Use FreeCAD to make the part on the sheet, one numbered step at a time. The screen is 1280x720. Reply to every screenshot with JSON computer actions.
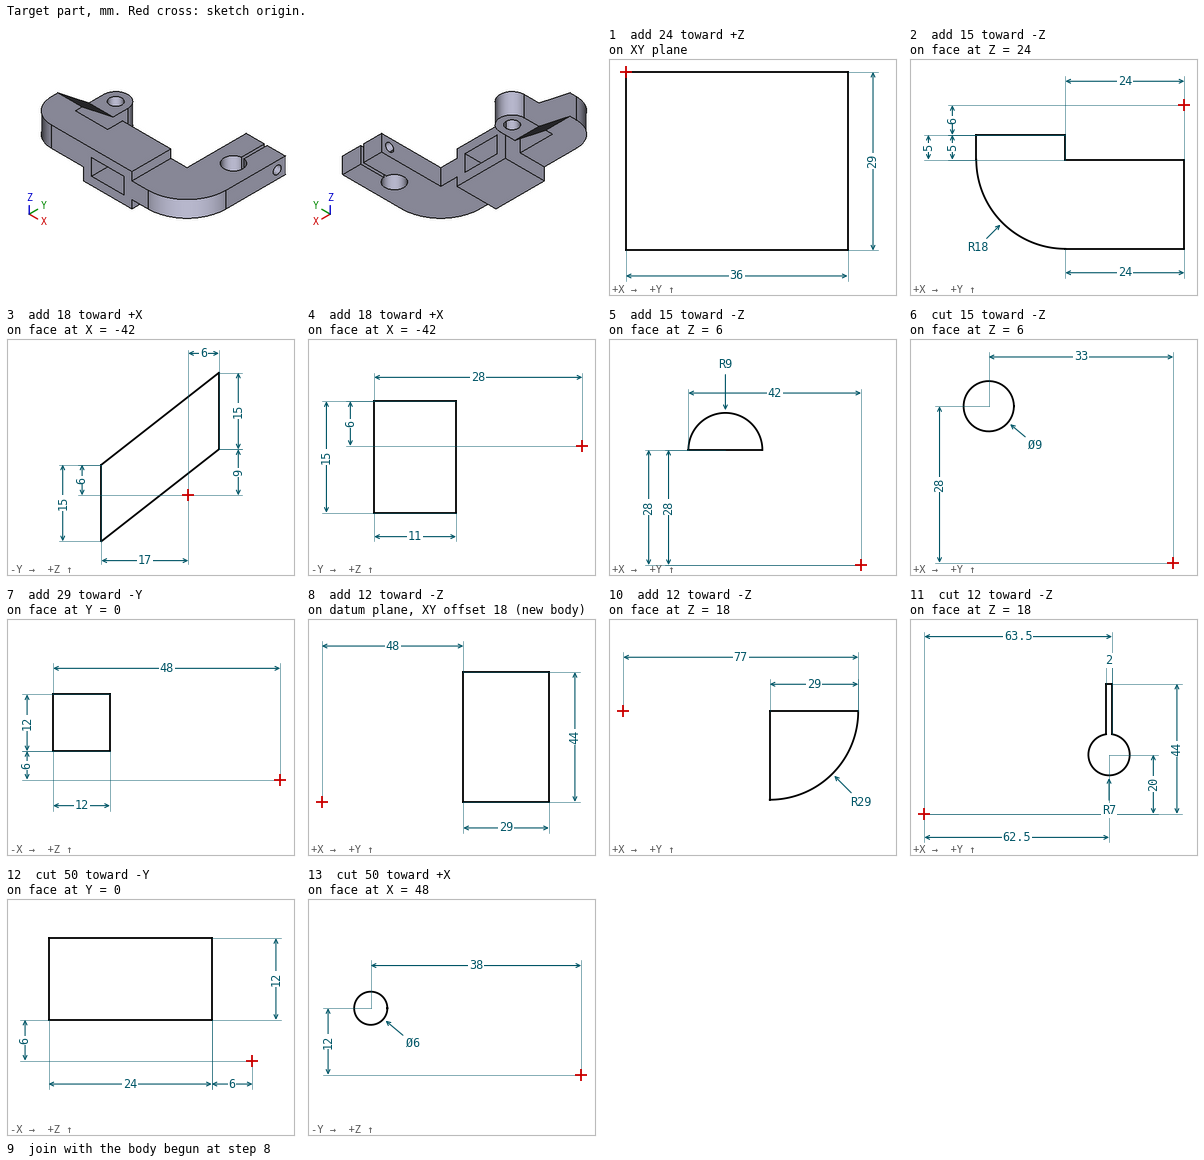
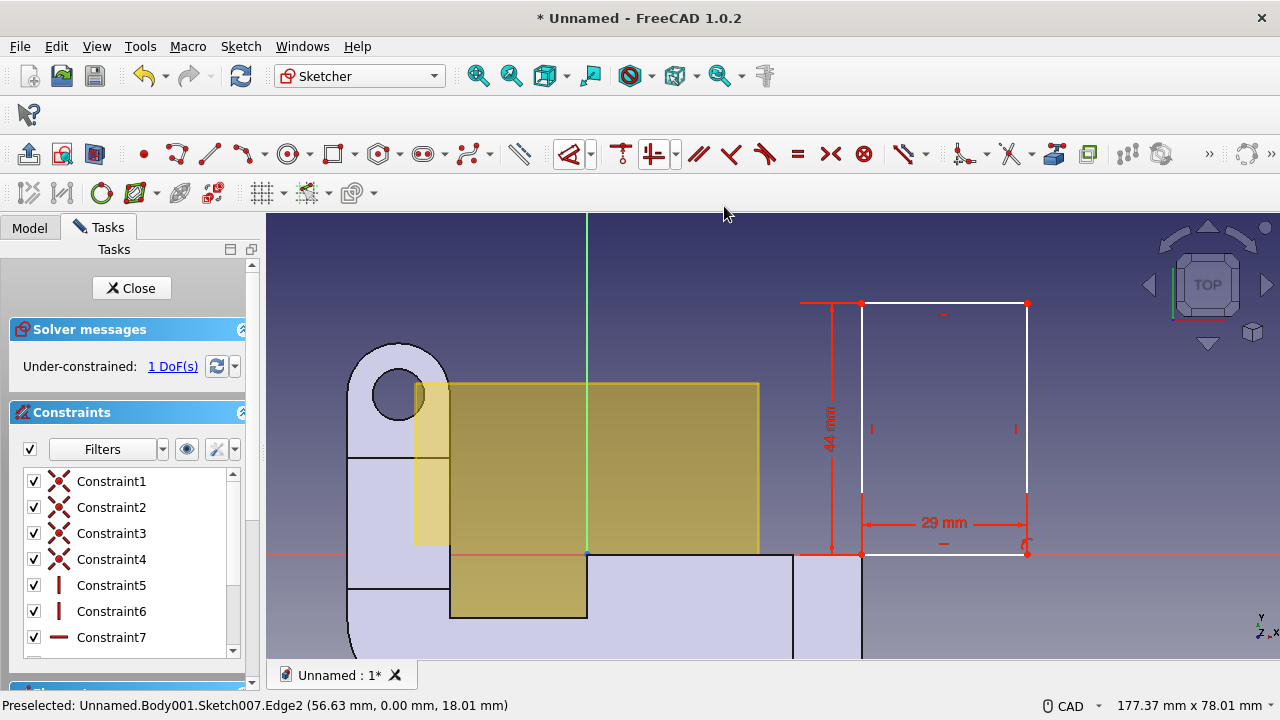
{"action": "left_click", "coordinate": [862, 303]}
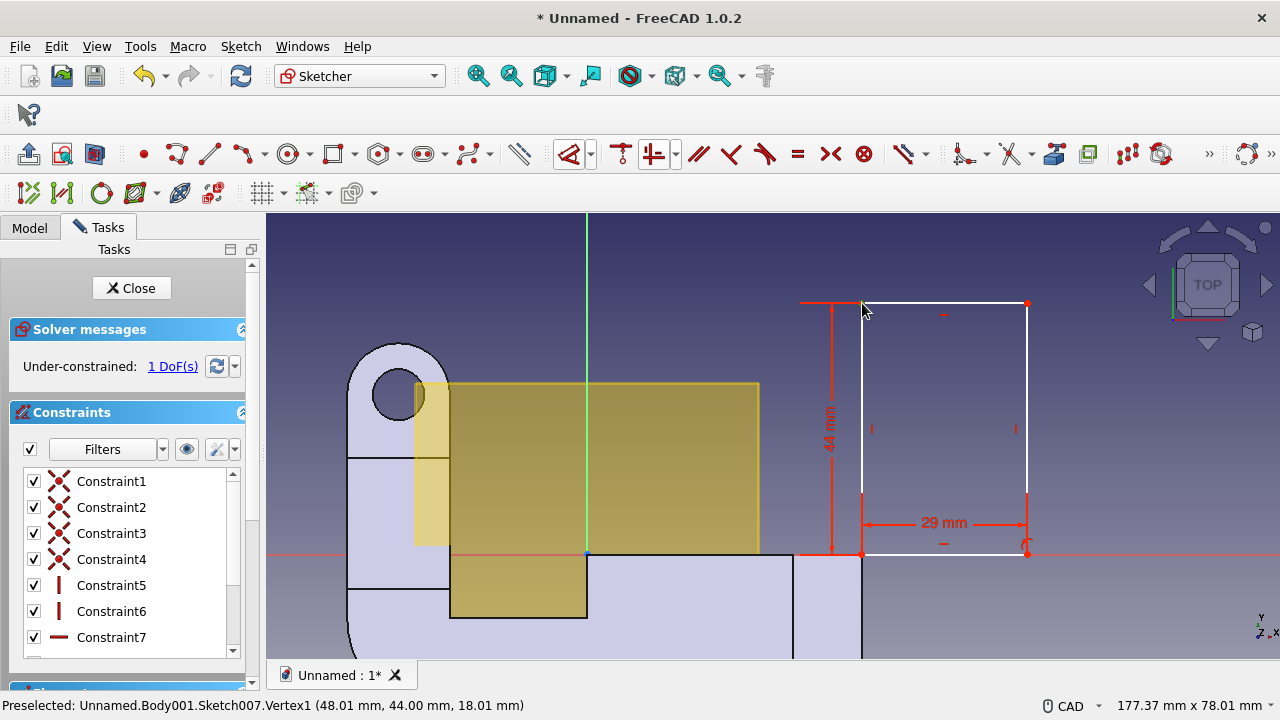
{"action": "key", "text": "l"}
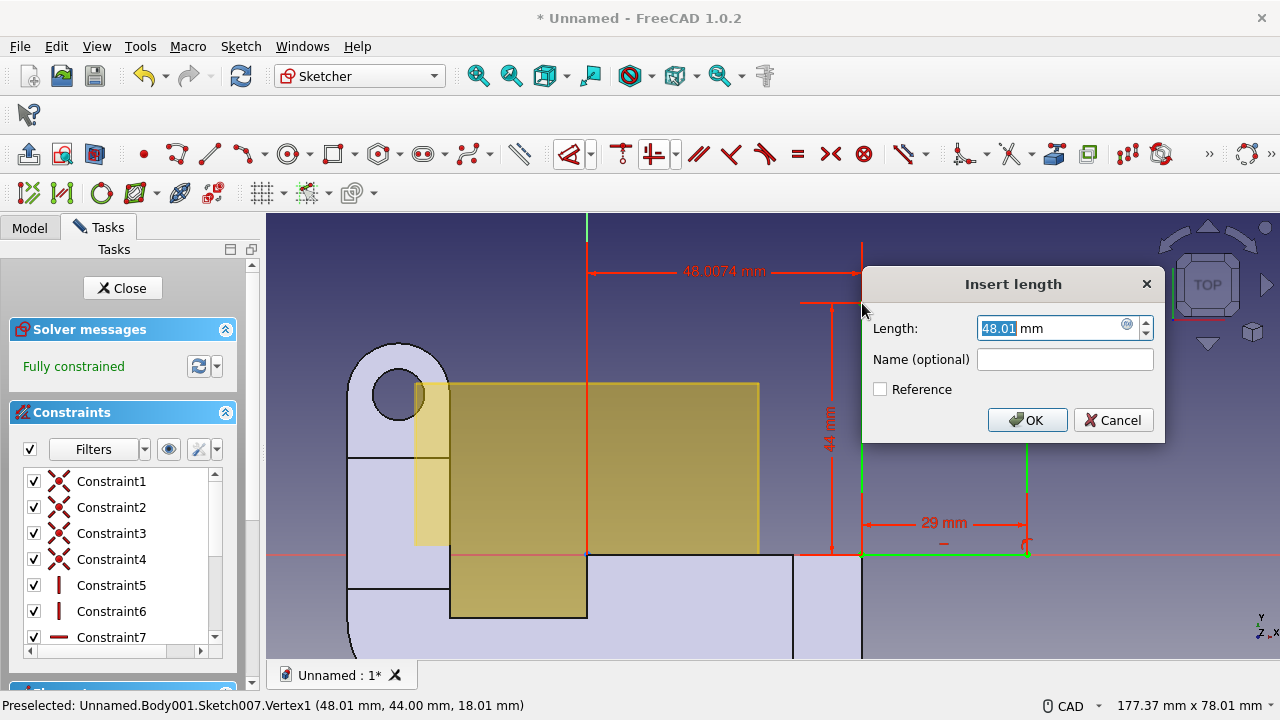
{"action": "type", "text": "48"}
{"action": "key", "text": "Return"}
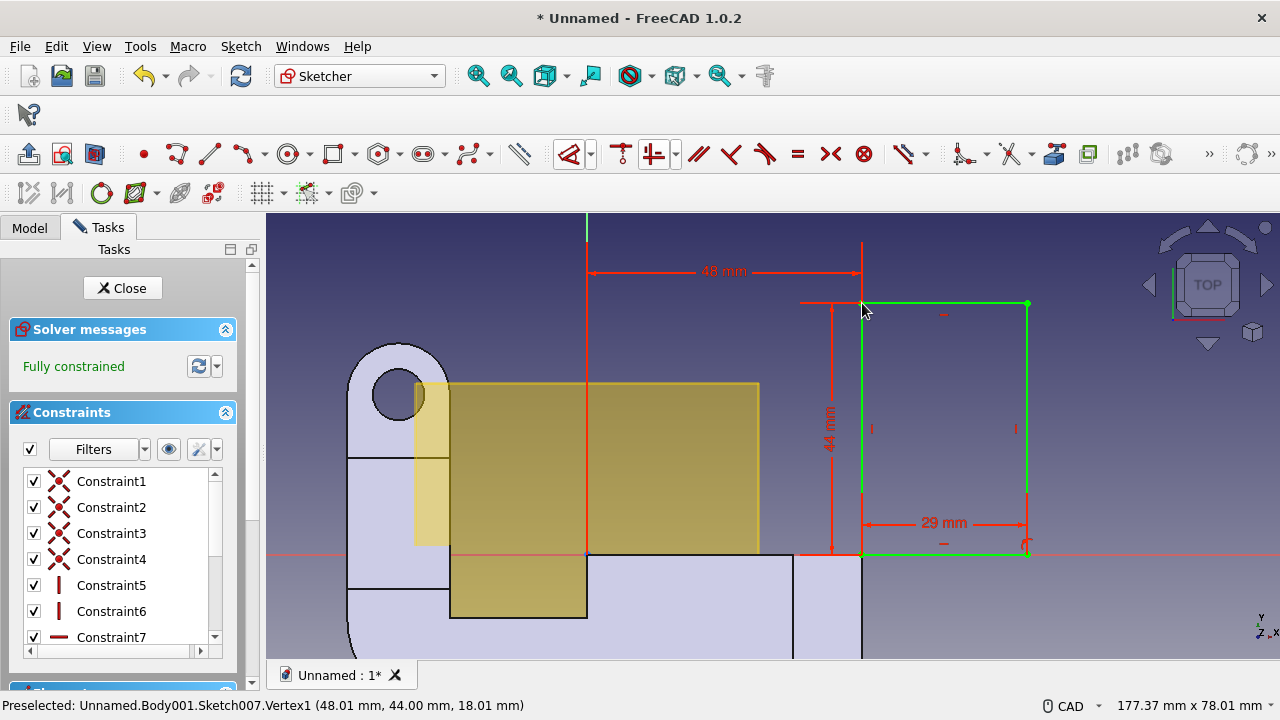
{"action": "left_click", "coordinate": [123, 288]}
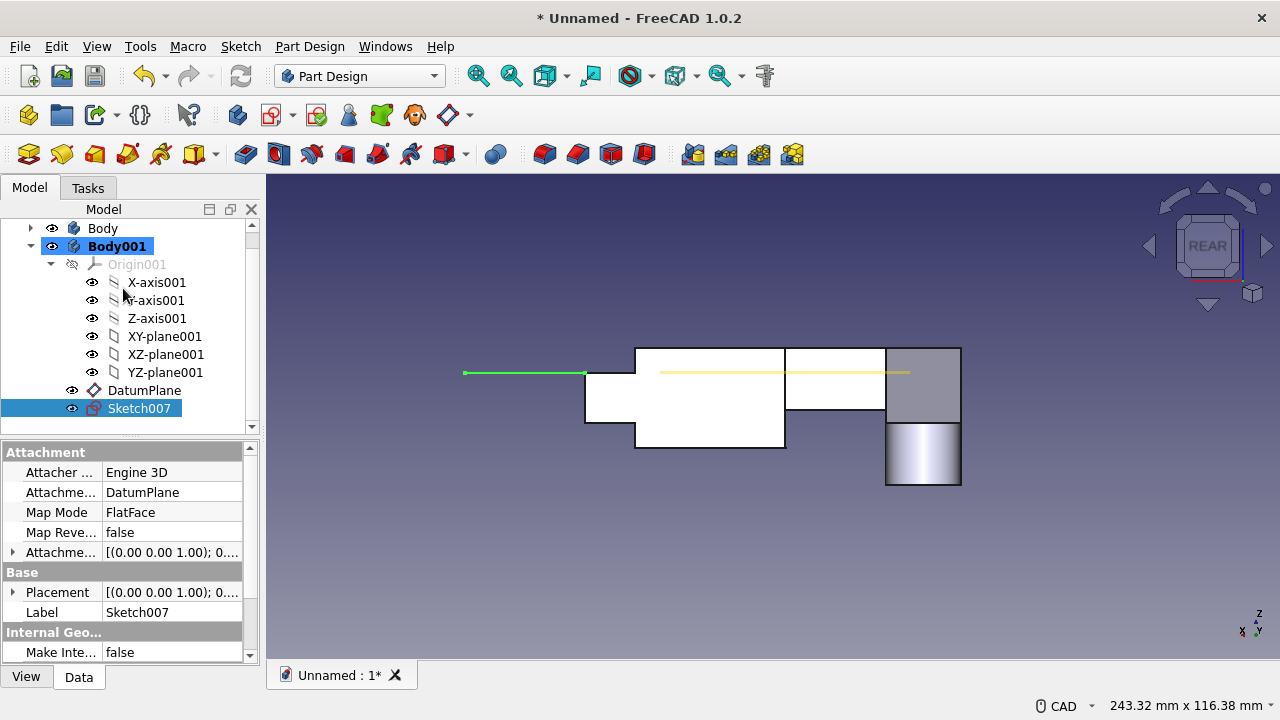
{"action": "left_click", "coordinate": [29, 154]}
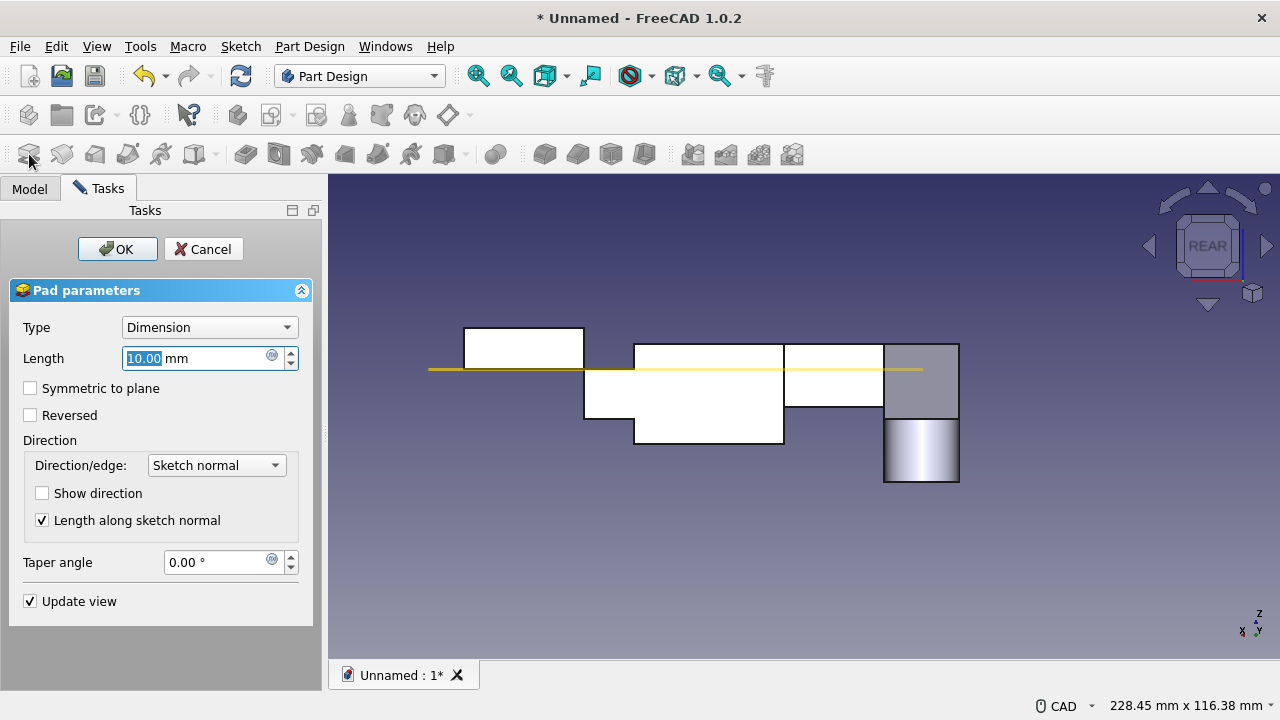
{"action": "type", "text": "12"}
{"action": "key", "text": "Tab"}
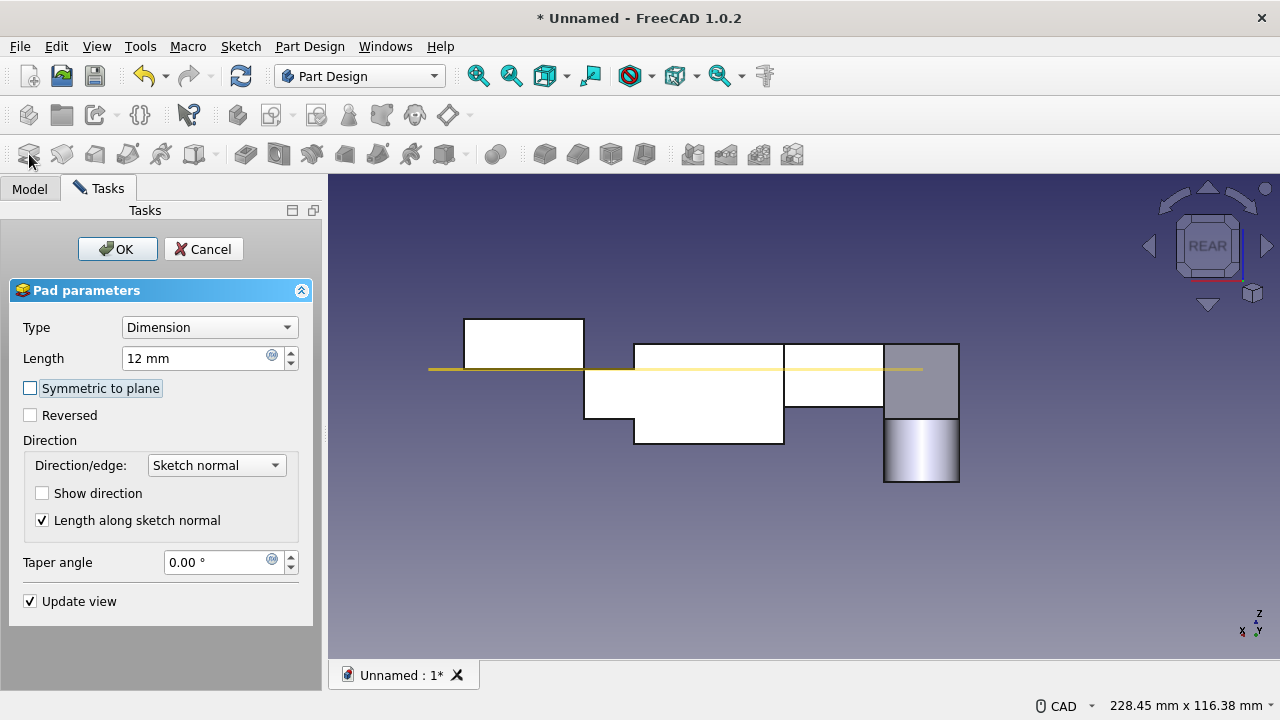
{"action": "left_click", "coordinate": [31, 415]}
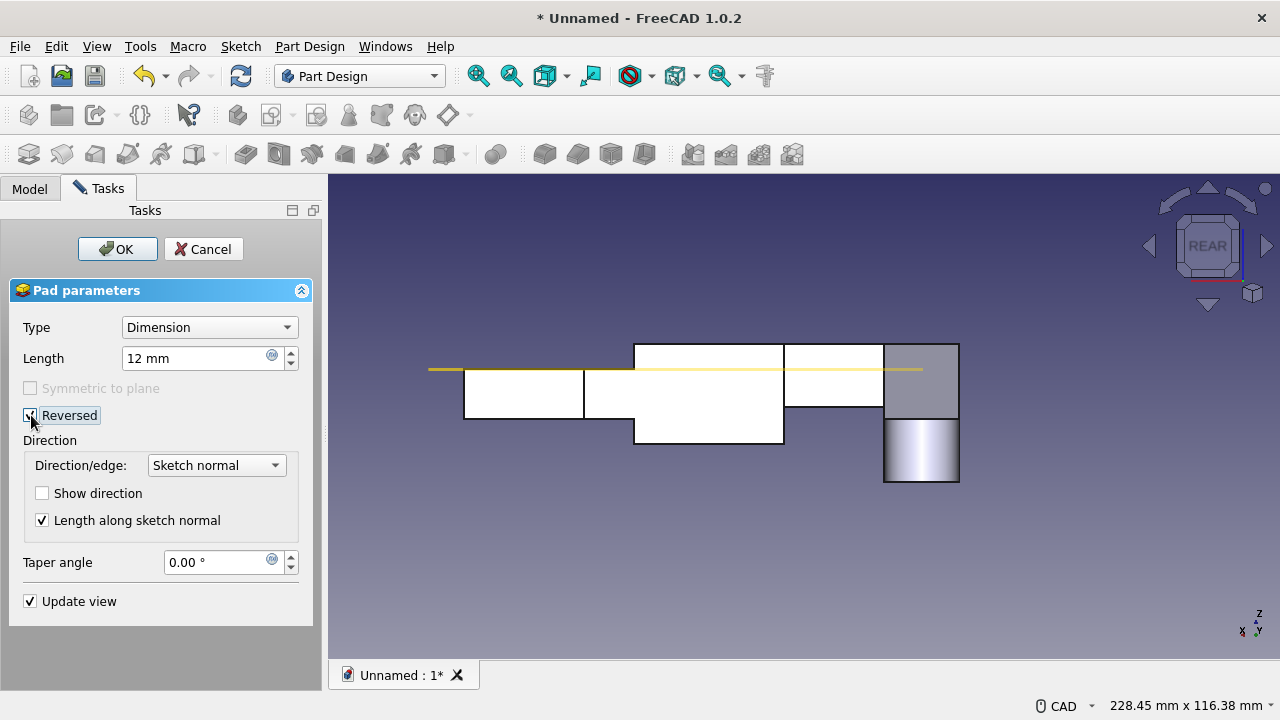
{"action": "left_click", "coordinate": [118, 249]}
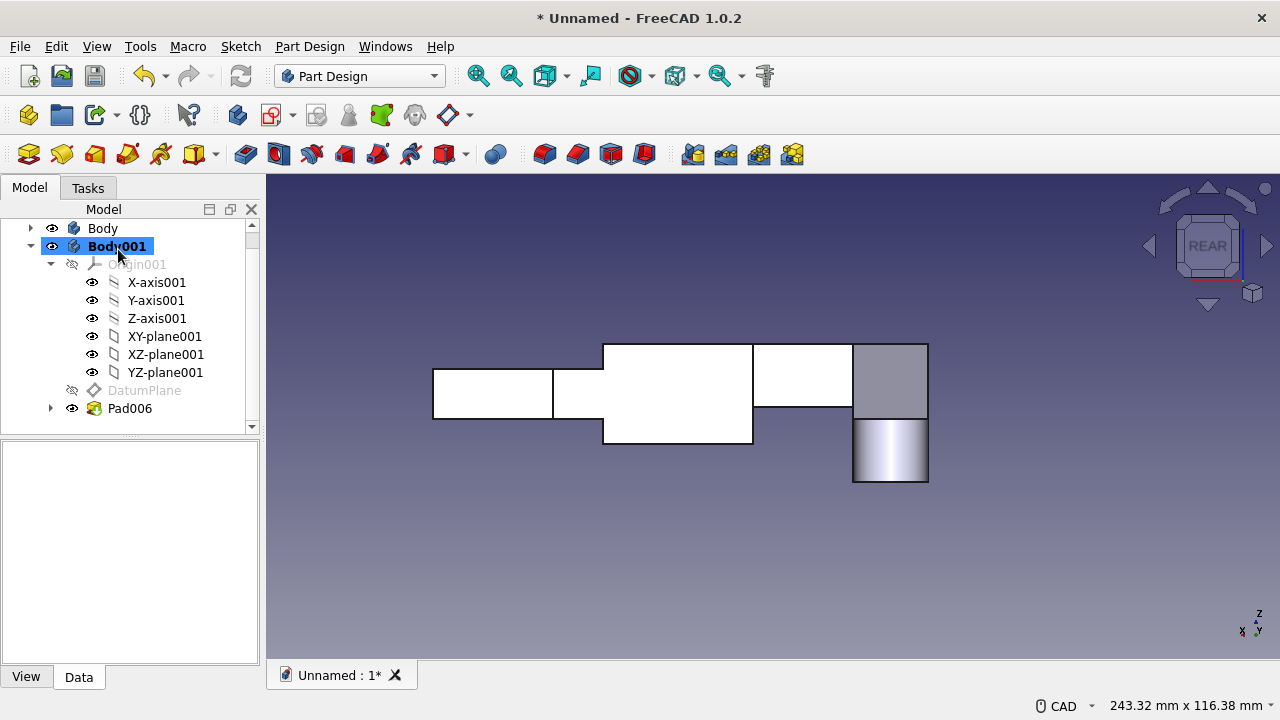
{"action": "left_click", "coordinate": [479, 76]}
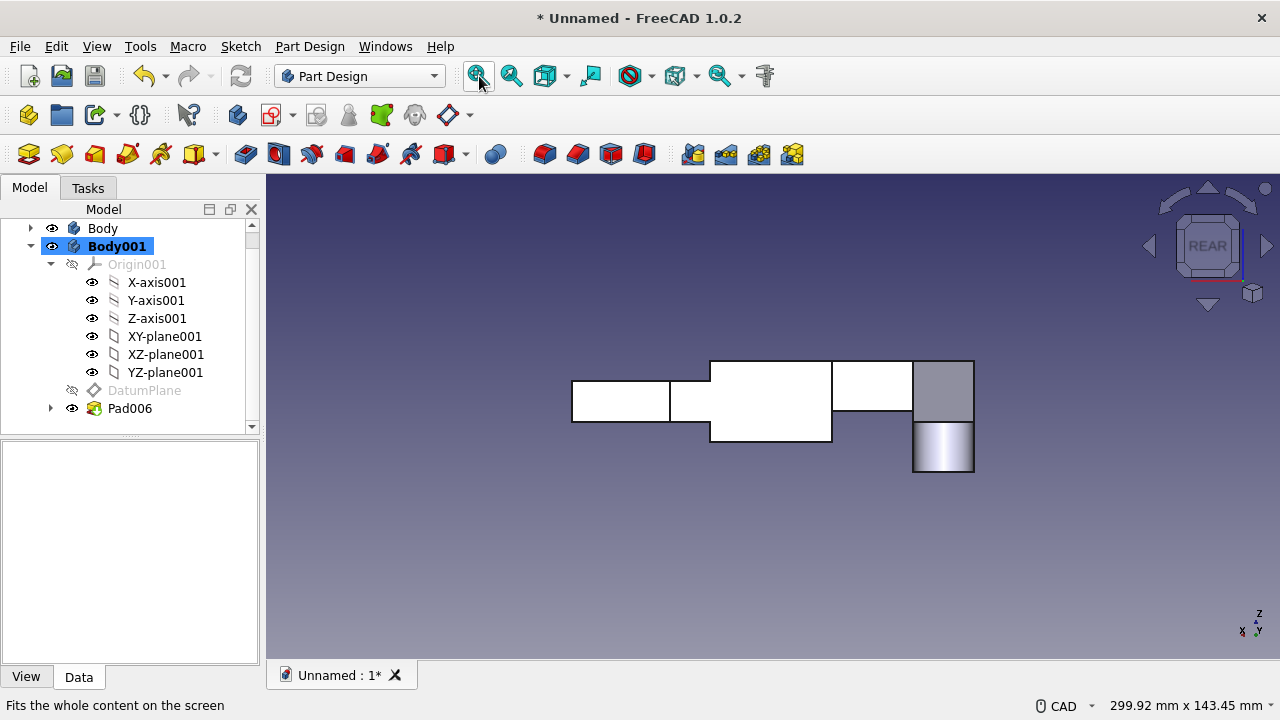
{"action": "double_click", "coordinate": [97, 228]}